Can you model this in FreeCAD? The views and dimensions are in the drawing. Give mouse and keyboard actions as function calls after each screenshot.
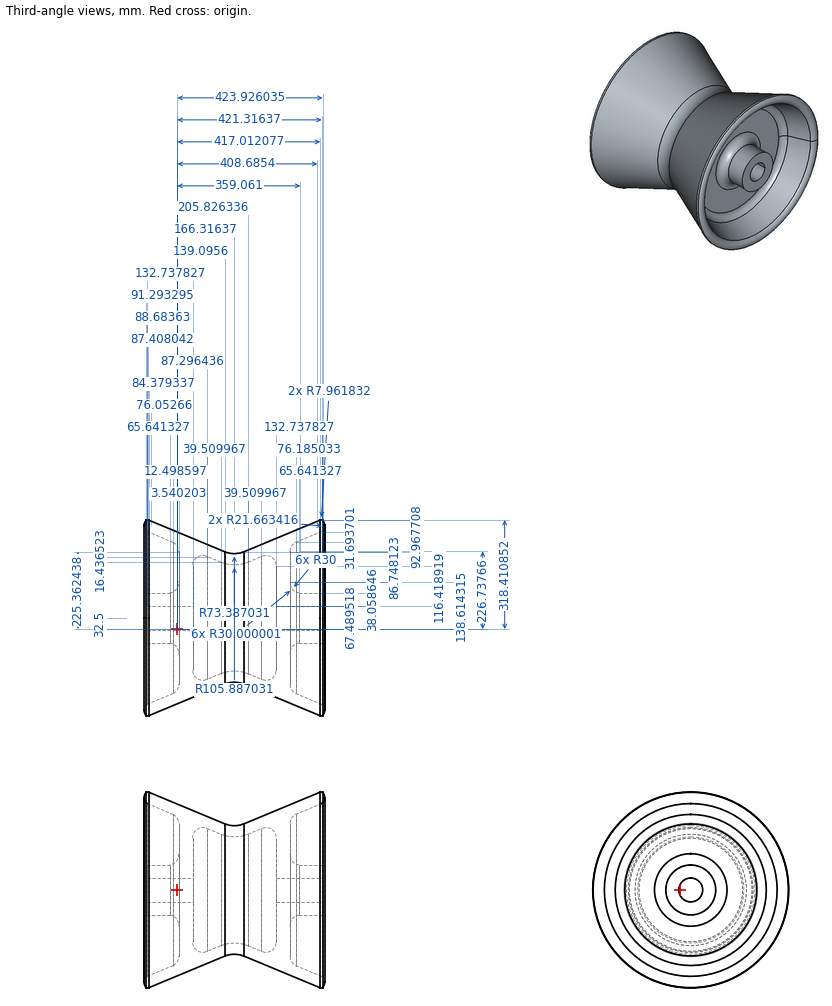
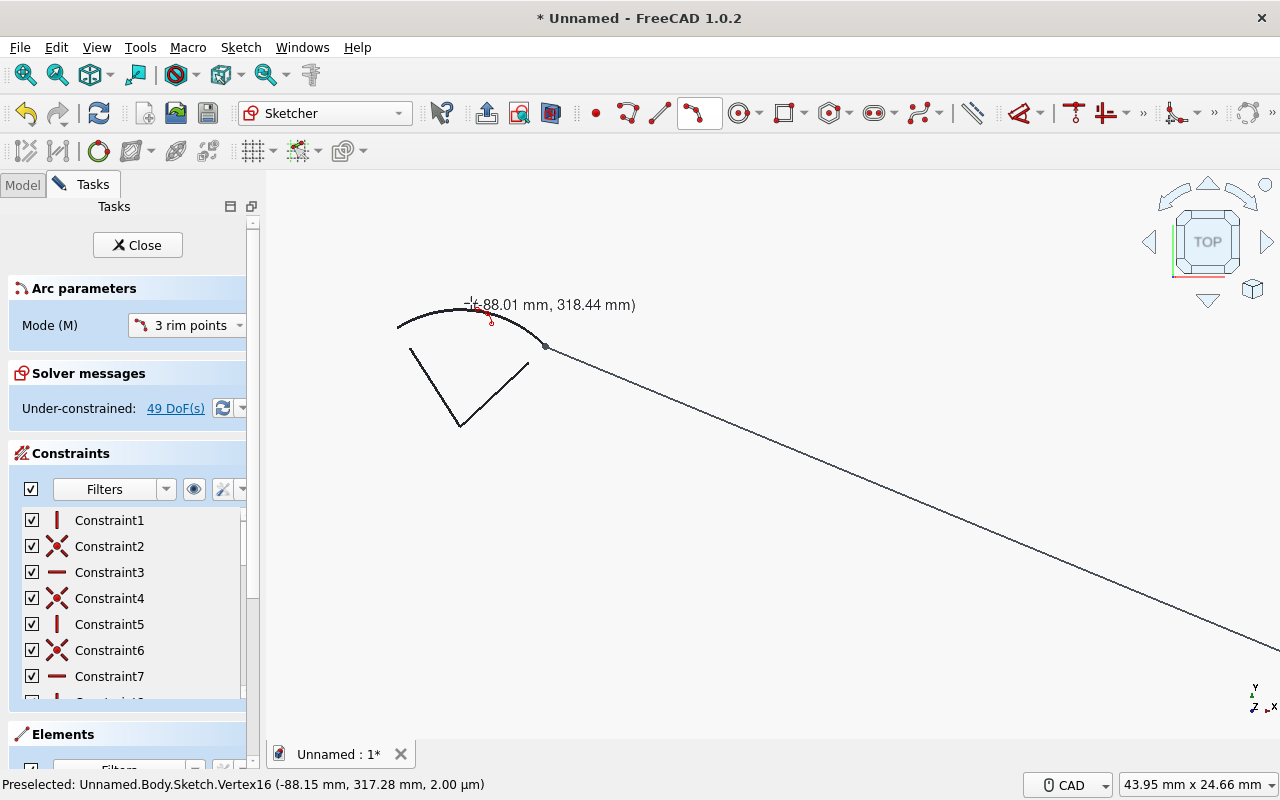
click(472, 297)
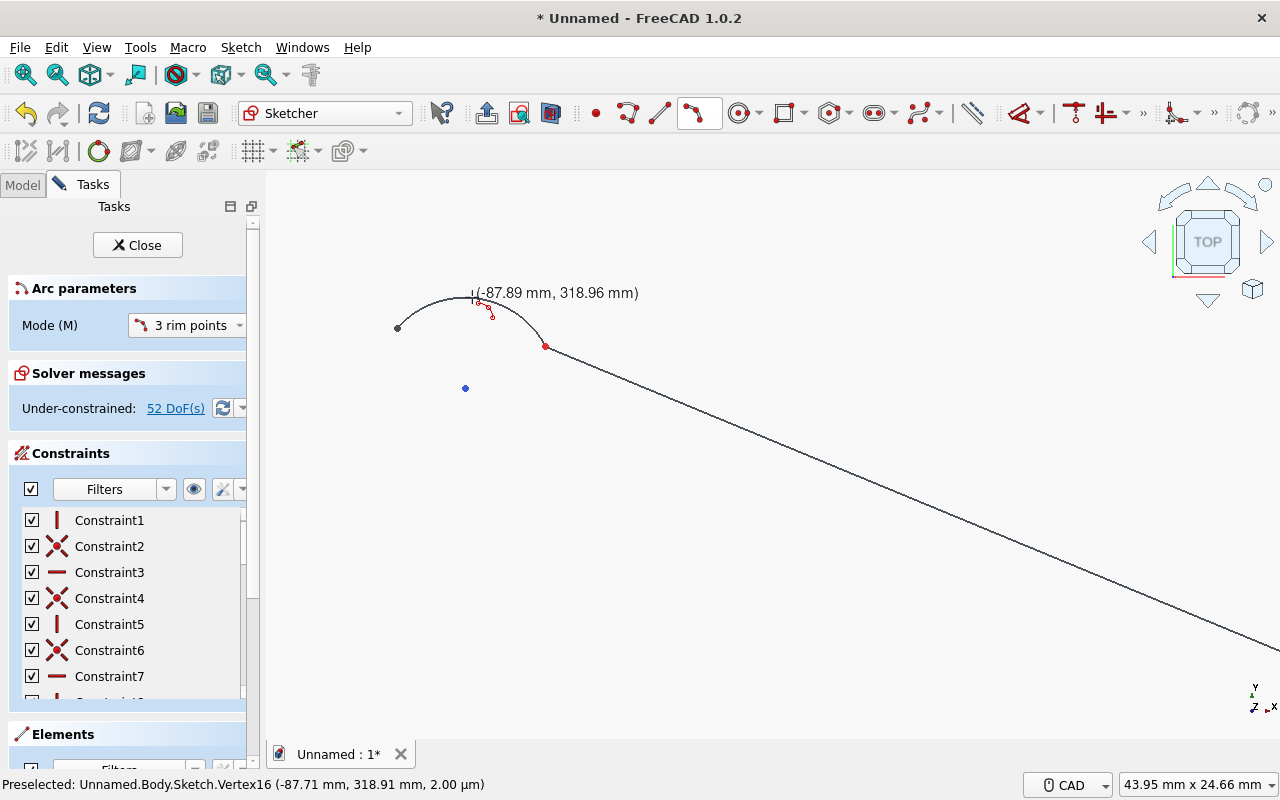
scroll(409, 270, down, 15)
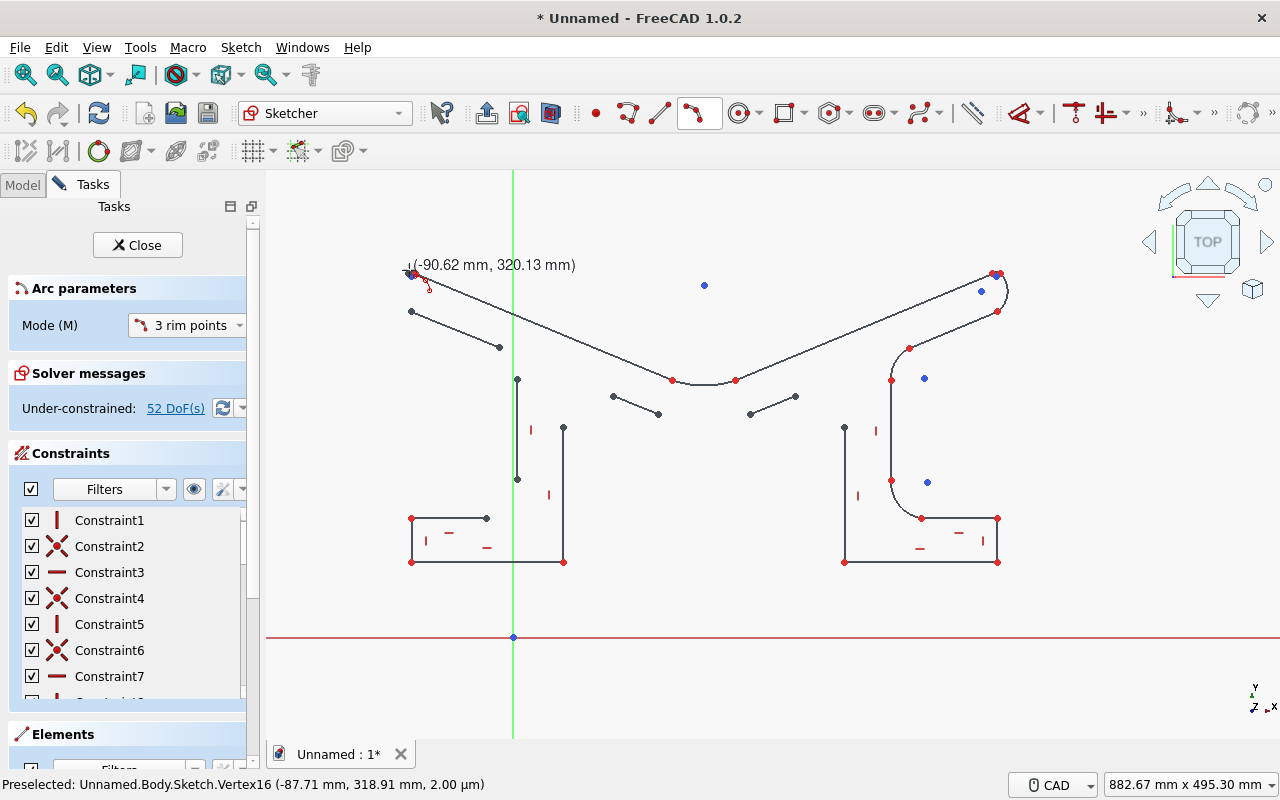
scroll(408, 273, up, 4)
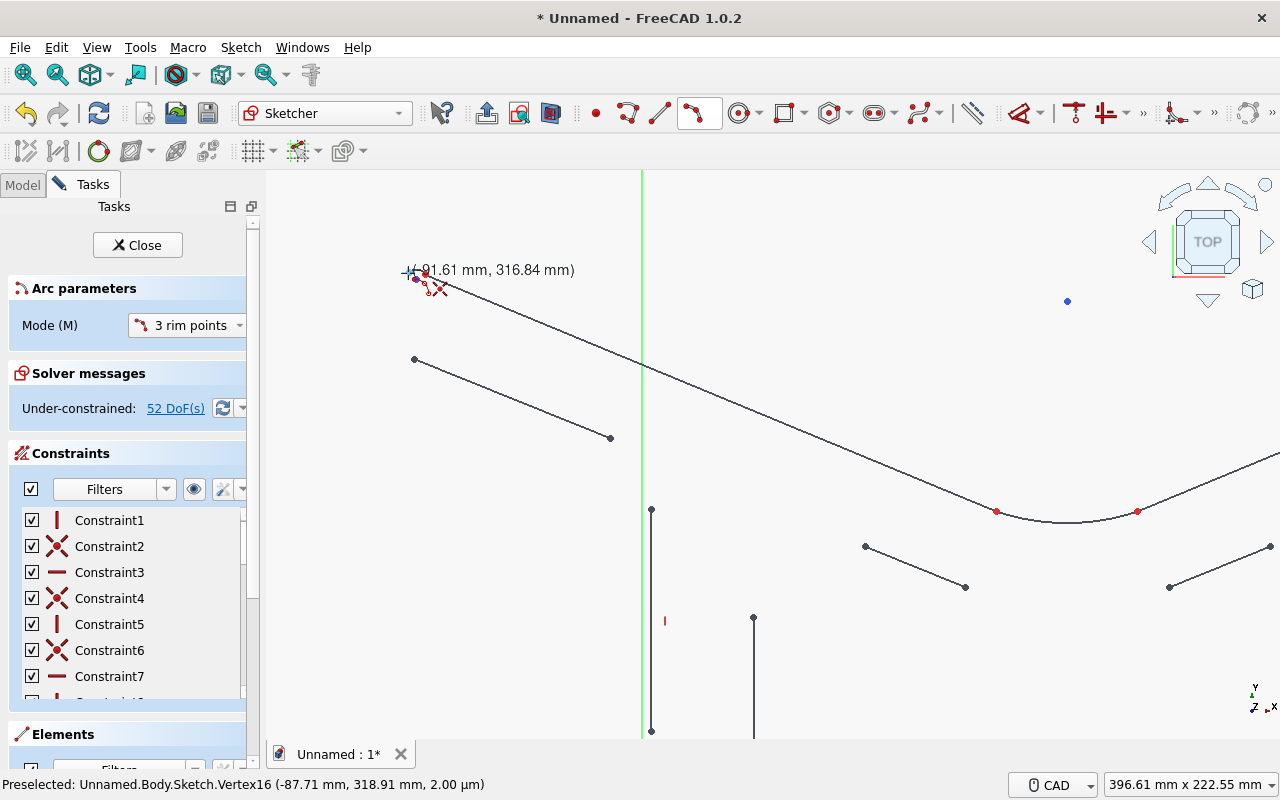
click(409, 273)
click(415, 359)
click(392, 316)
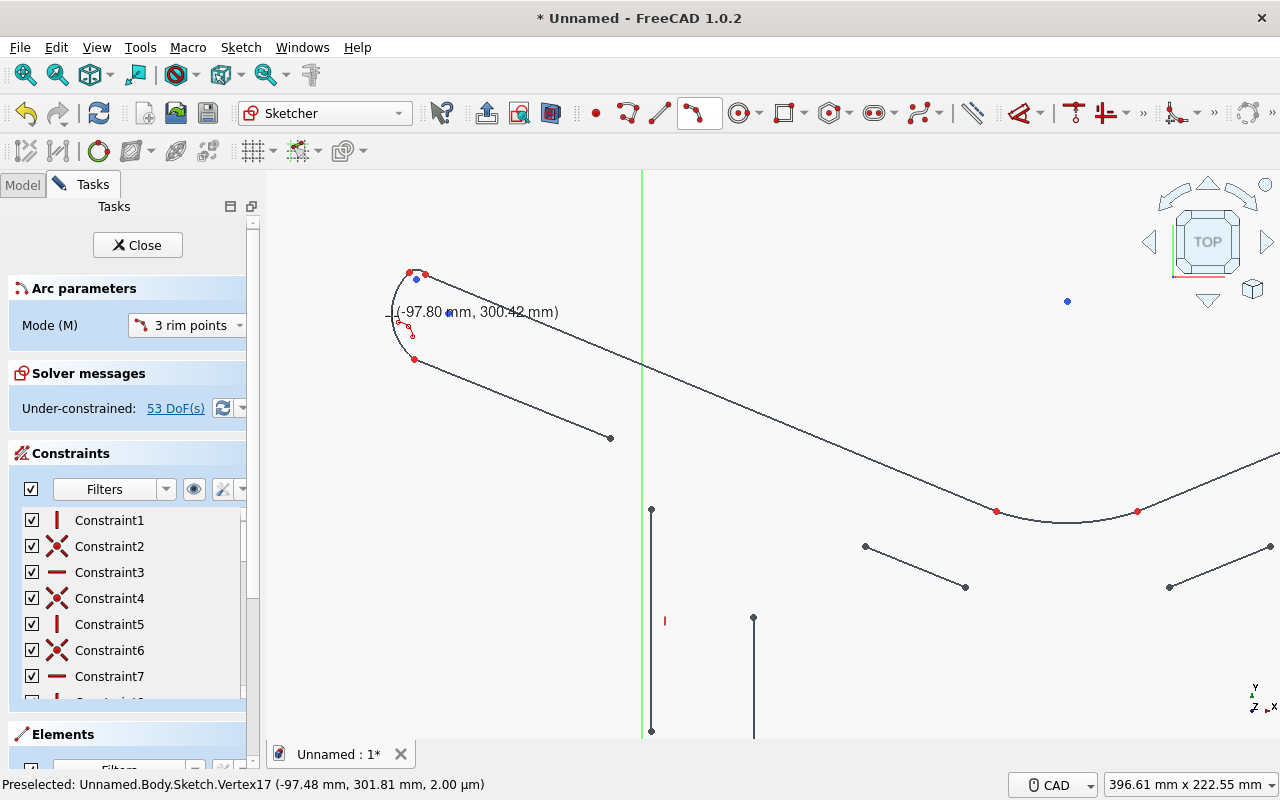
click(611, 438)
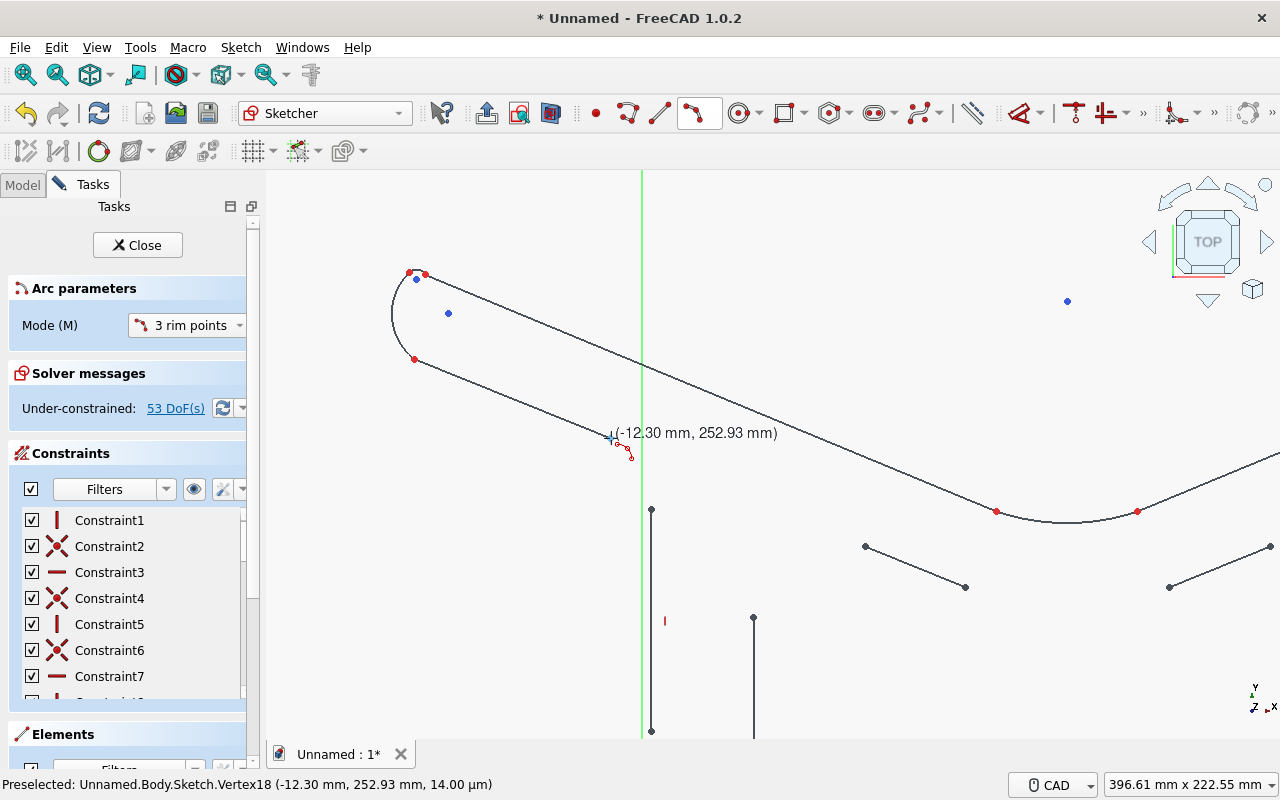
scroll(651, 509, up, 3)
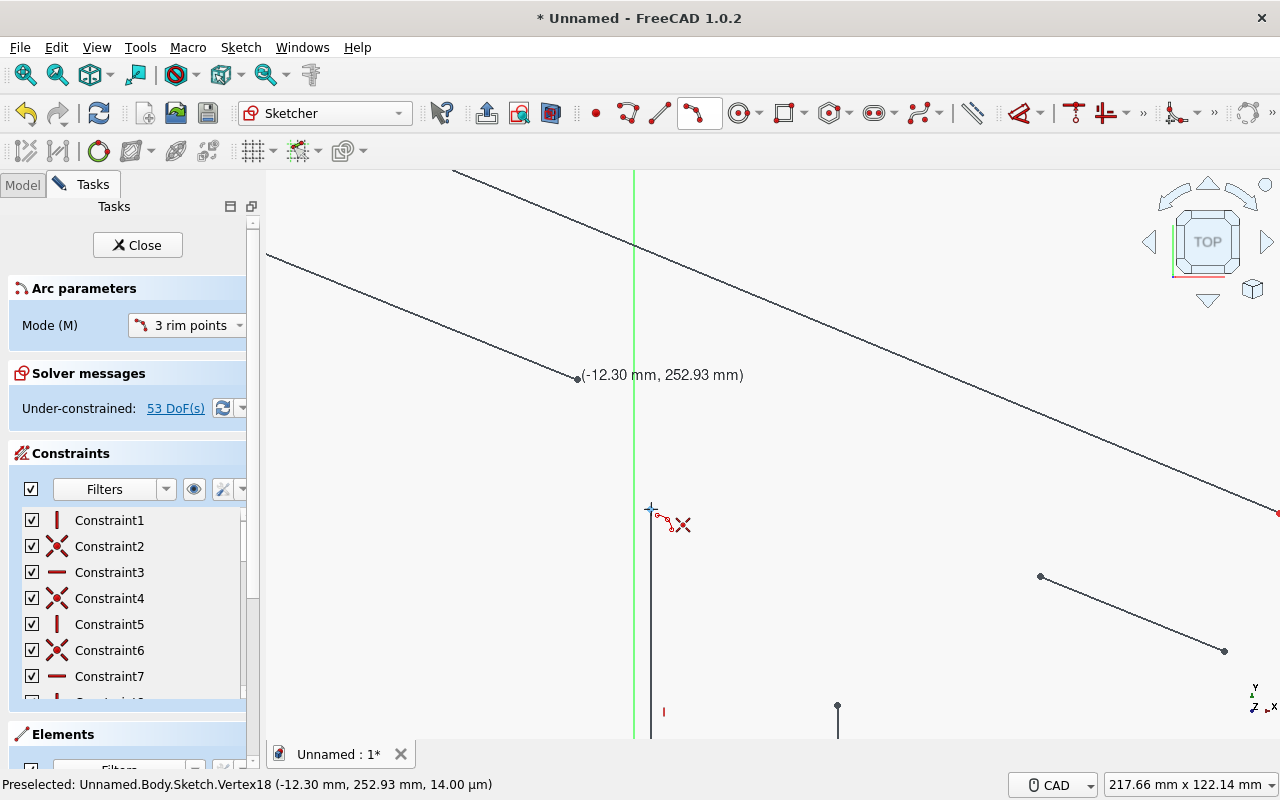
click(651, 509)
click(614, 407)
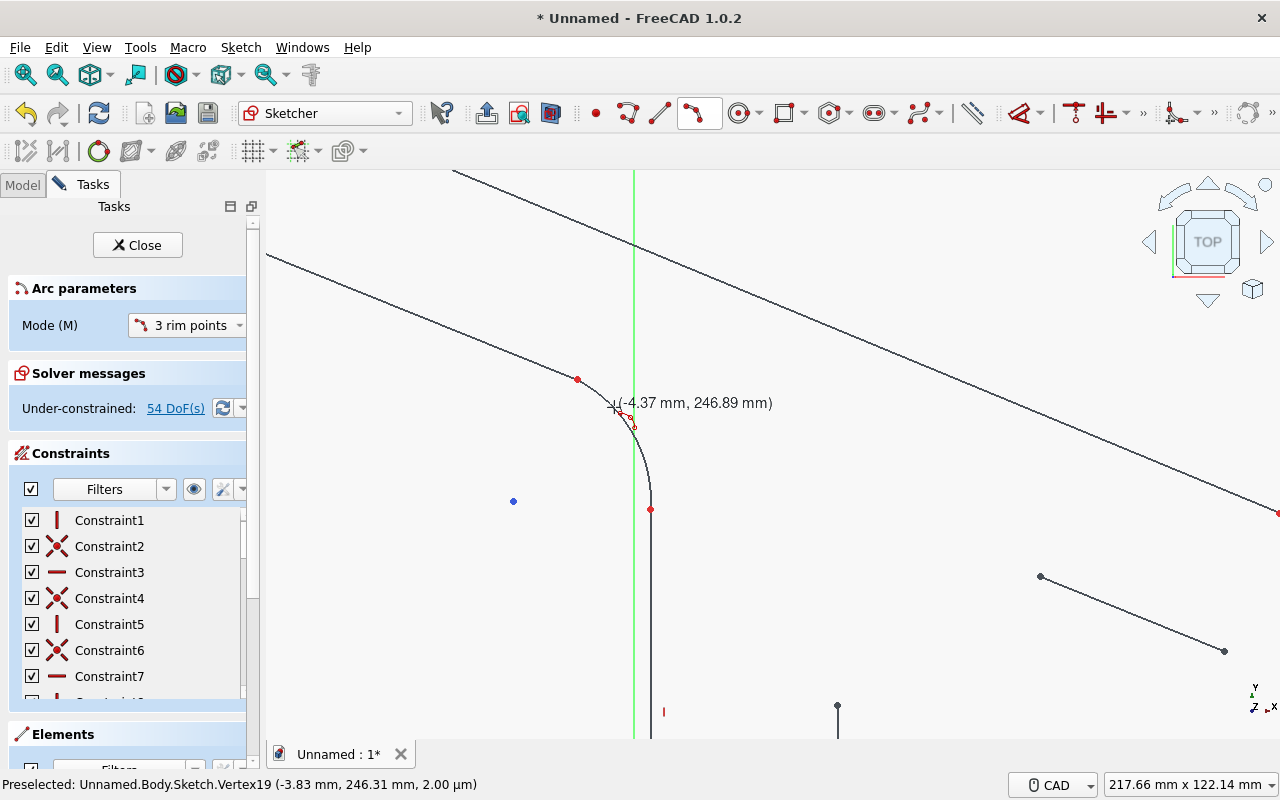
scroll(526, 363, down, 8)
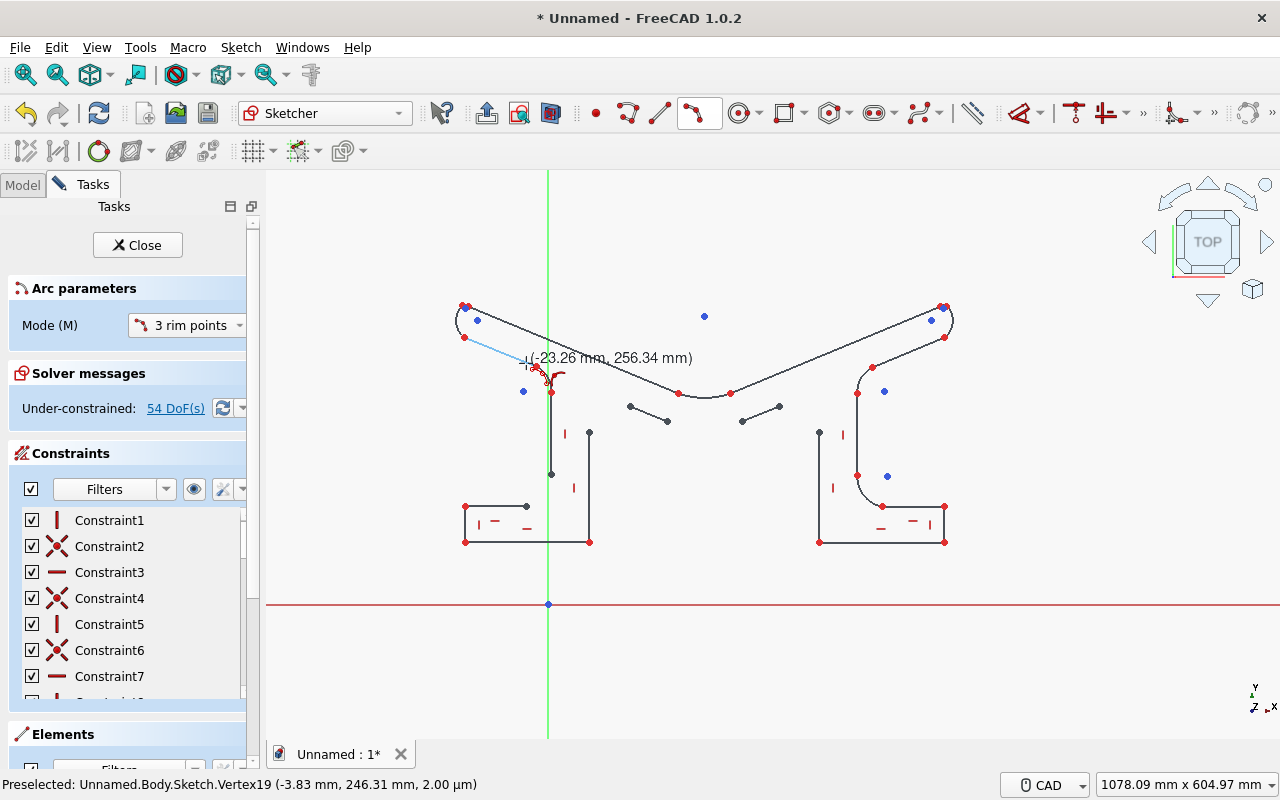
scroll(551, 474, up, 8)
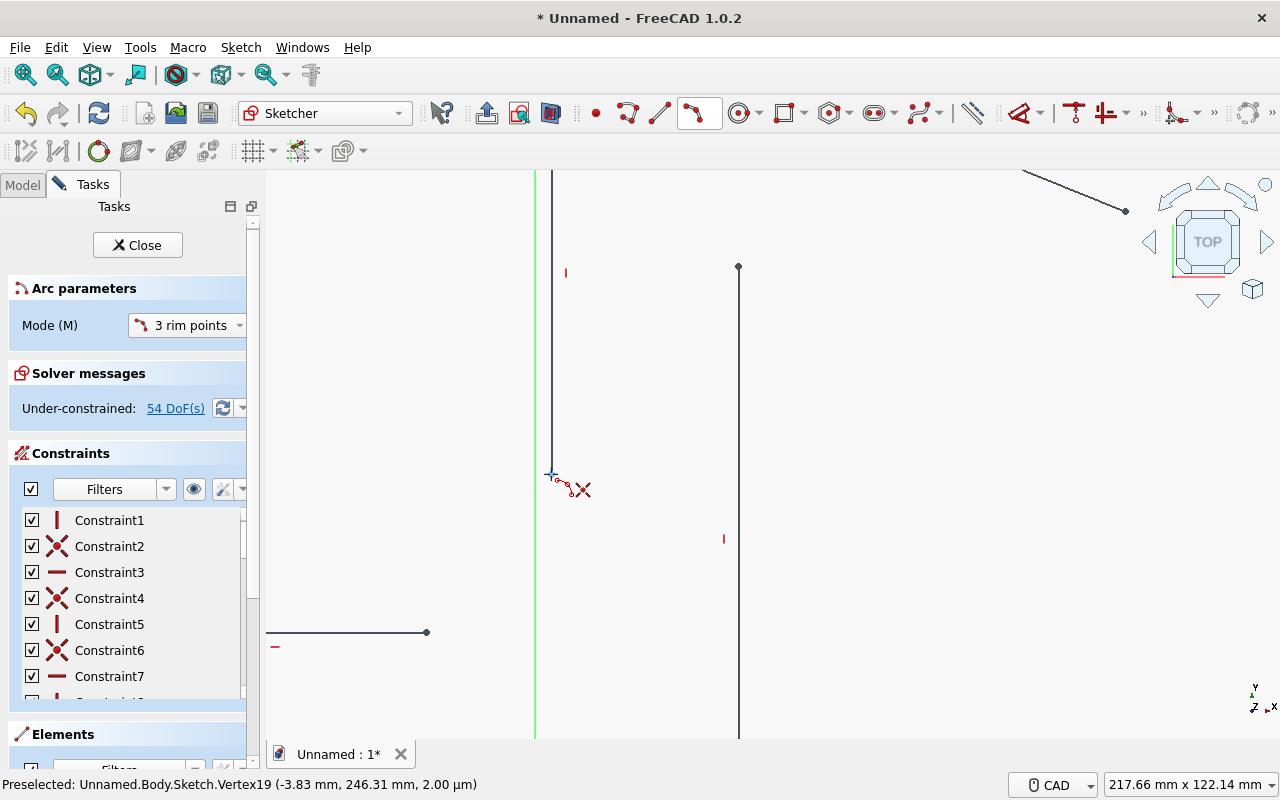
click(552, 474)